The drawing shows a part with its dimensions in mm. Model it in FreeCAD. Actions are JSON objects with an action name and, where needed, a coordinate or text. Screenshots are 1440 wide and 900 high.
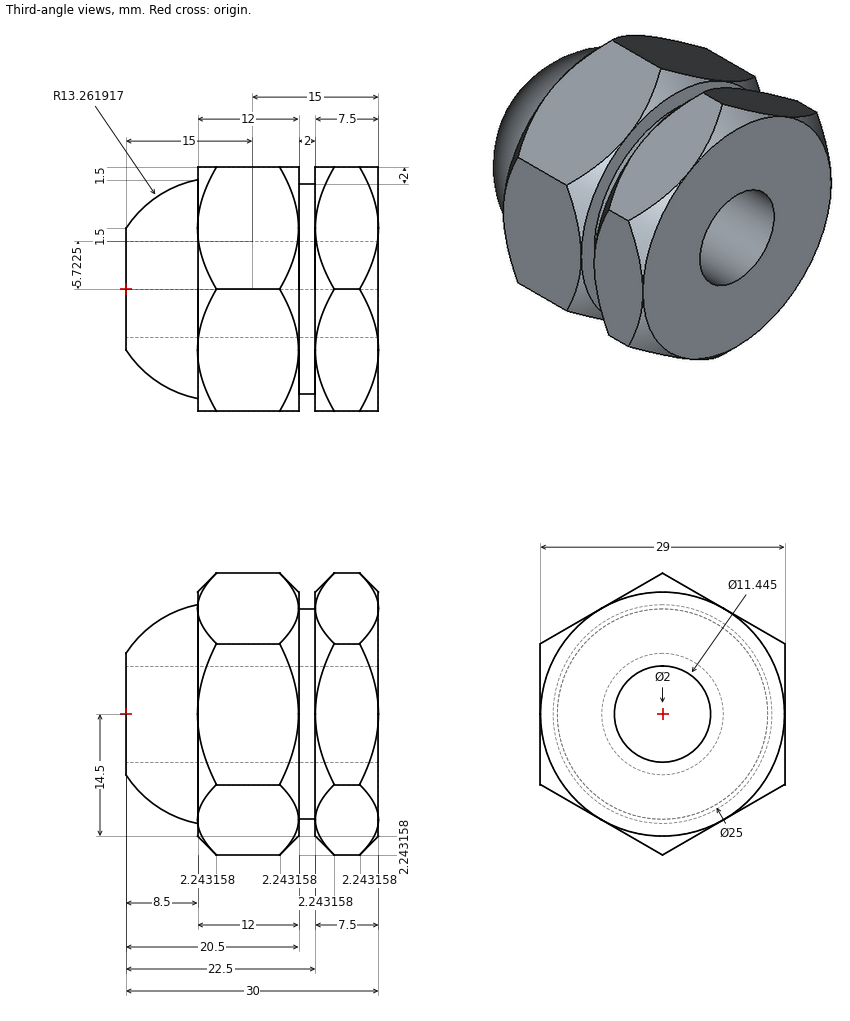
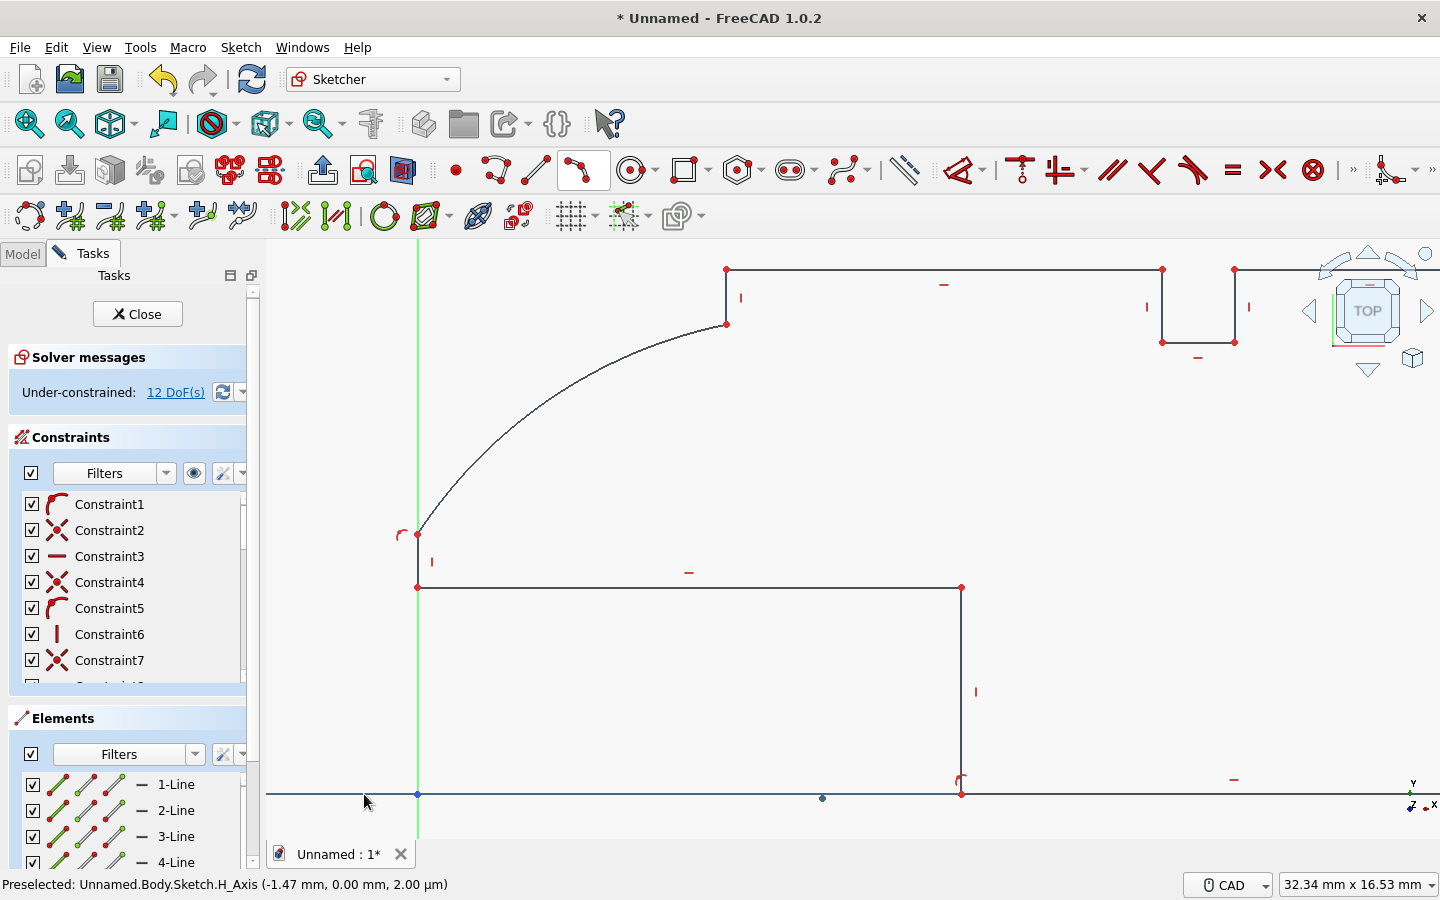
{"action": "left_click", "coordinate": [1020, 170]}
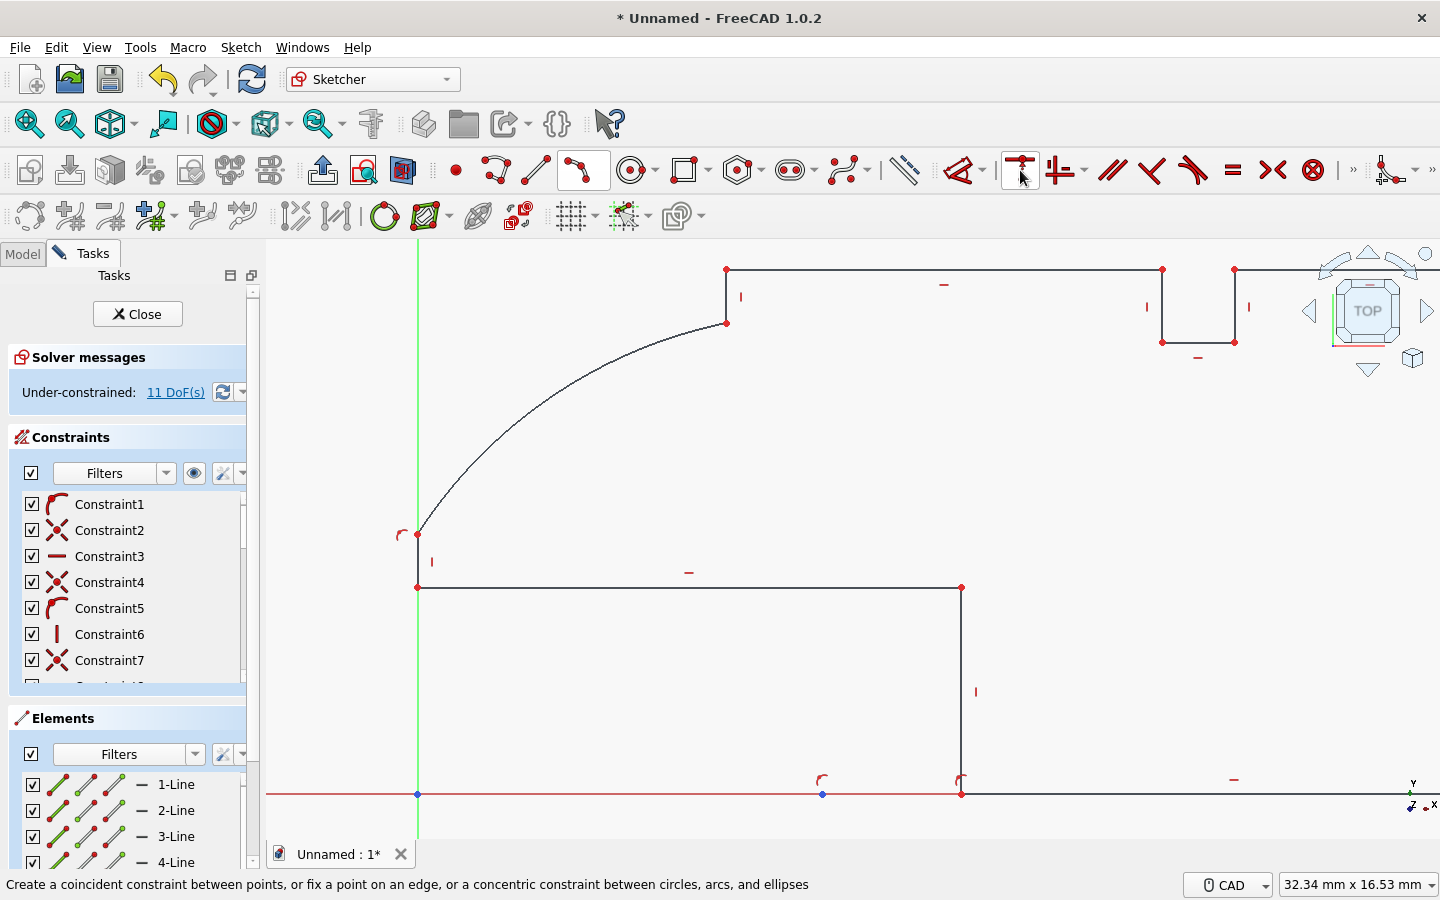
{"action": "left_click", "coordinate": [617, 359]}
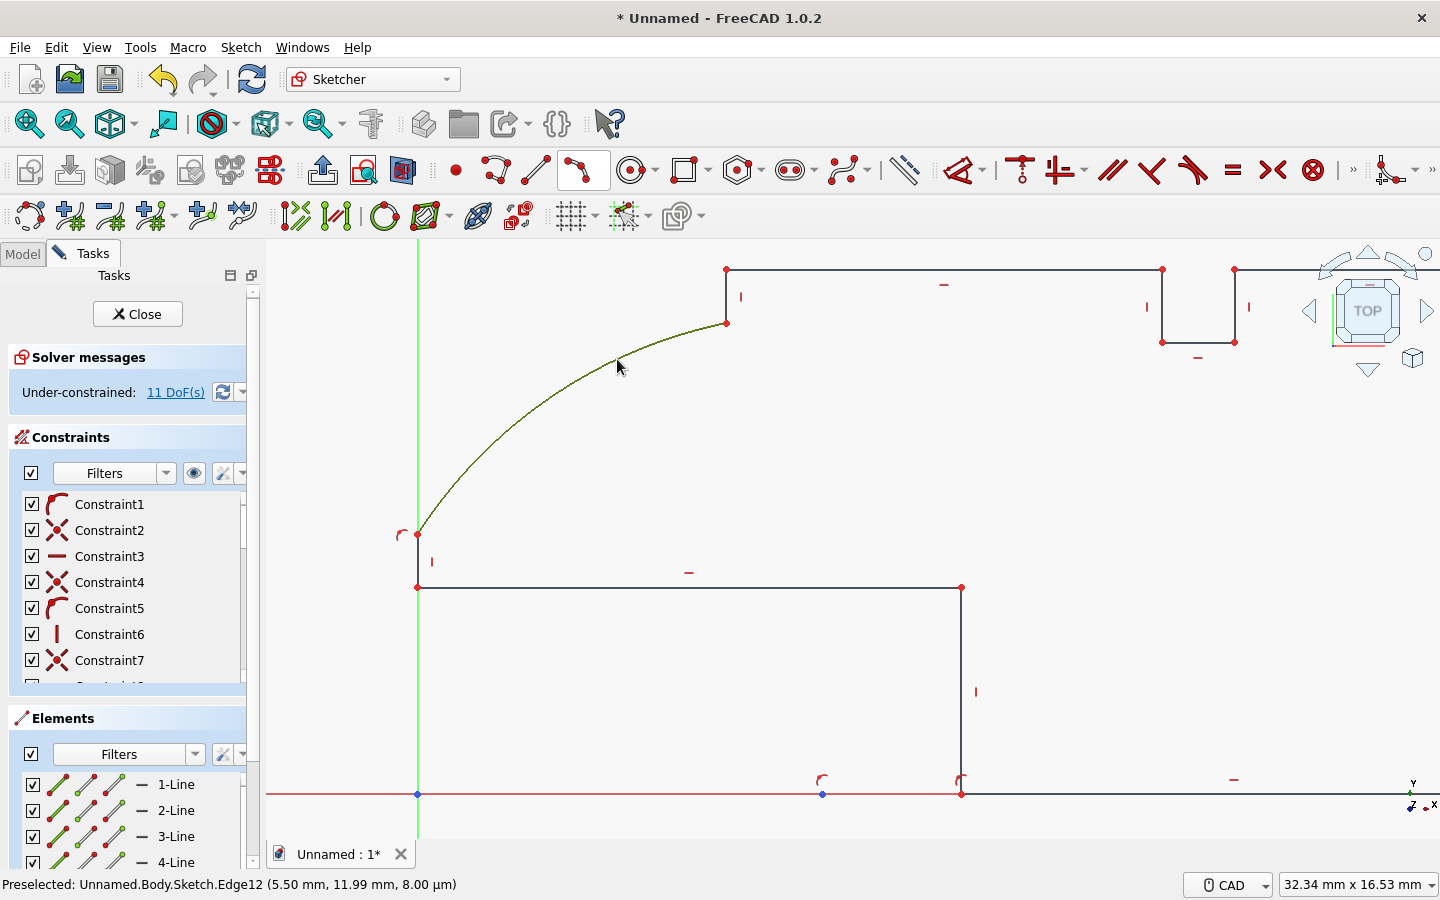
{"action": "key", "text": "k r"}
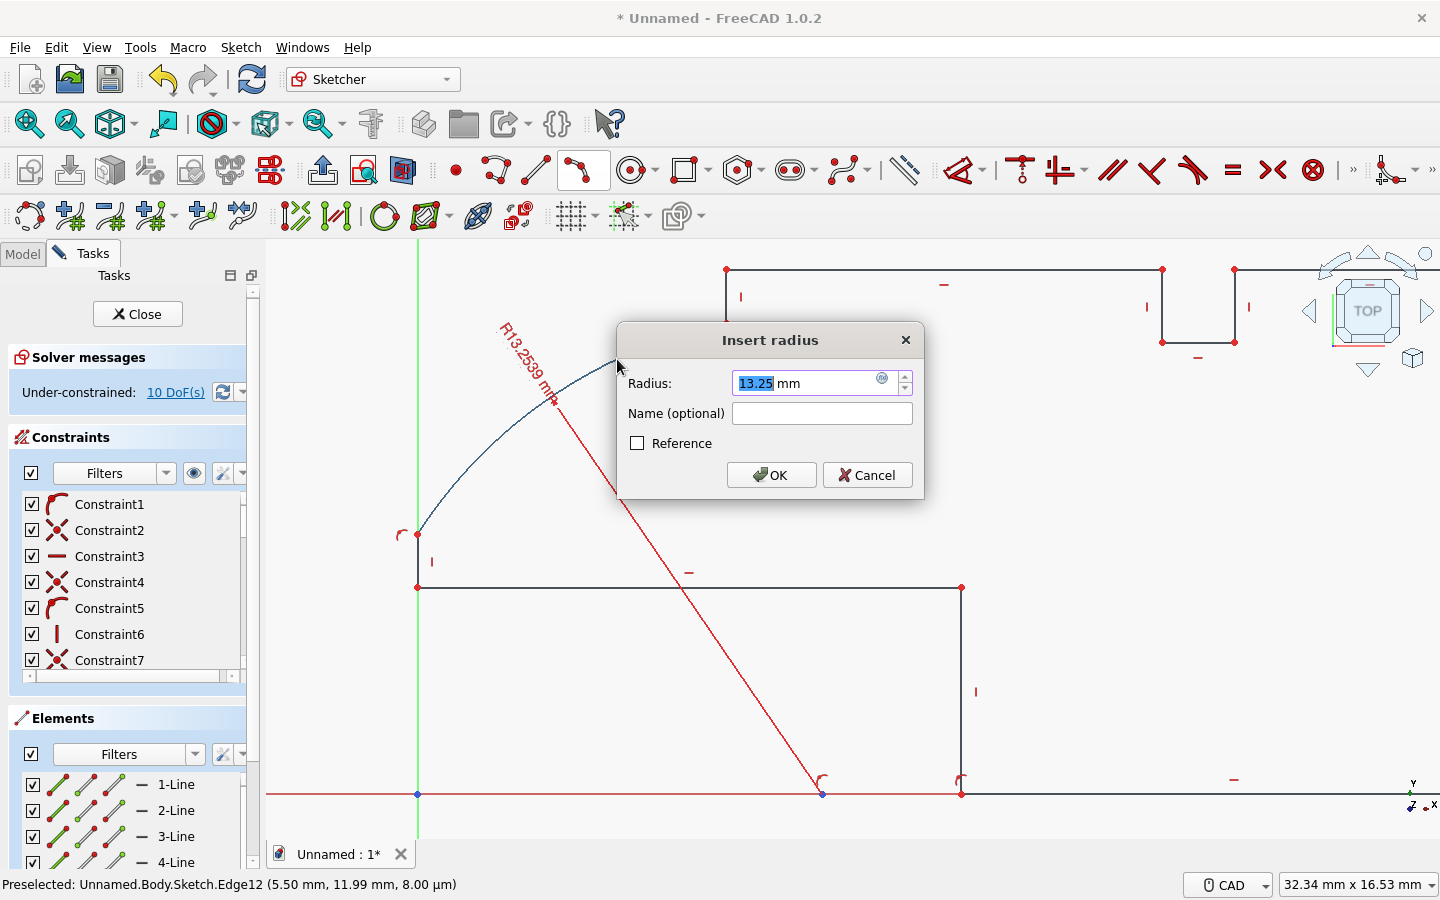
{"action": "type", "text": "13.261917"}
{"action": "key", "text": "Return"}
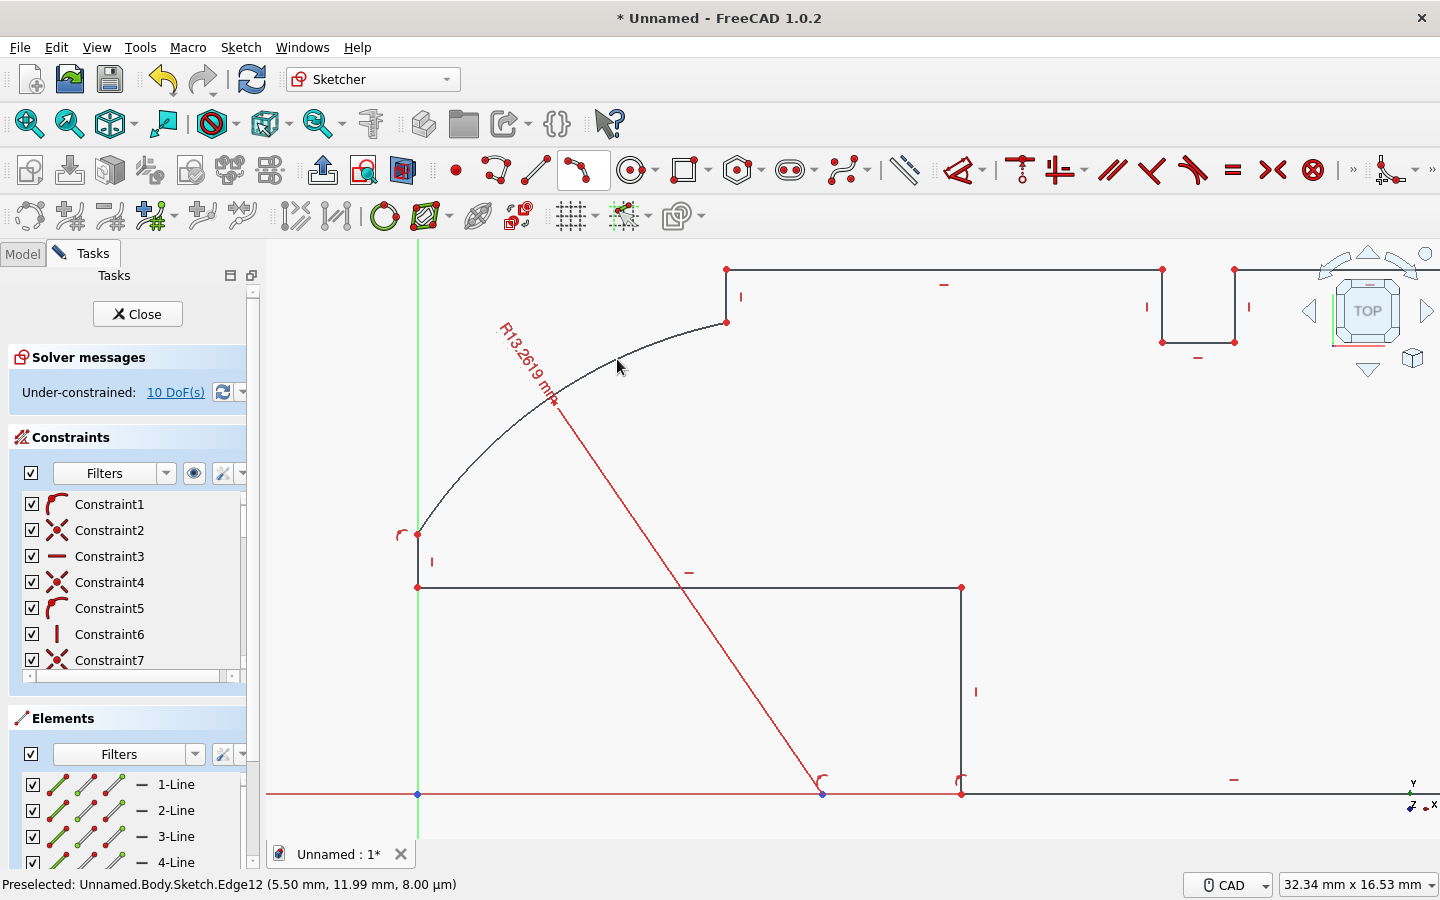
{"action": "left_click", "coordinate": [1235, 292]}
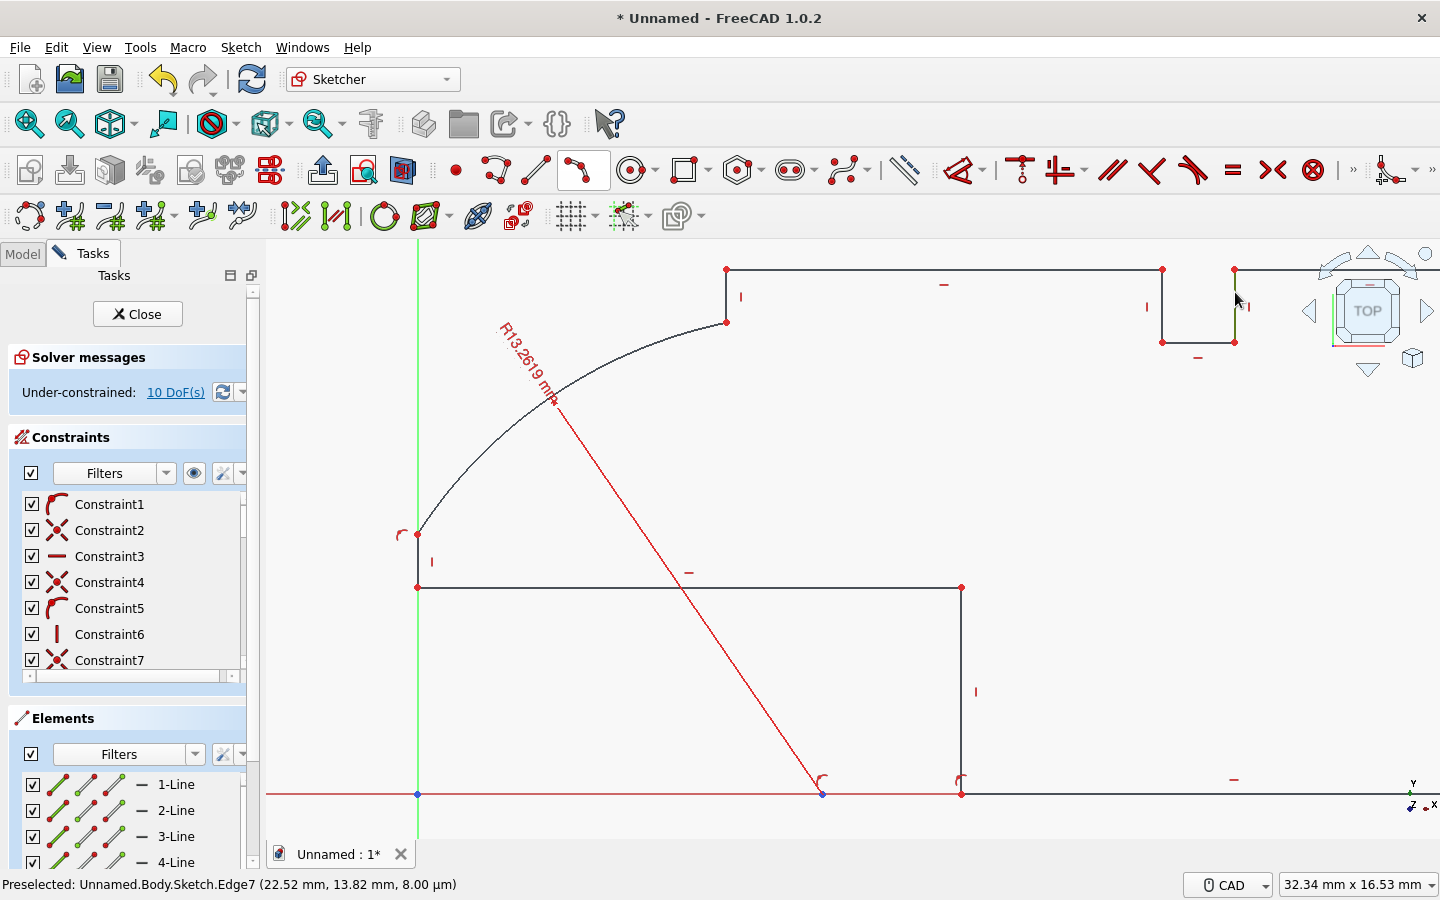
{"action": "key", "text": "i"}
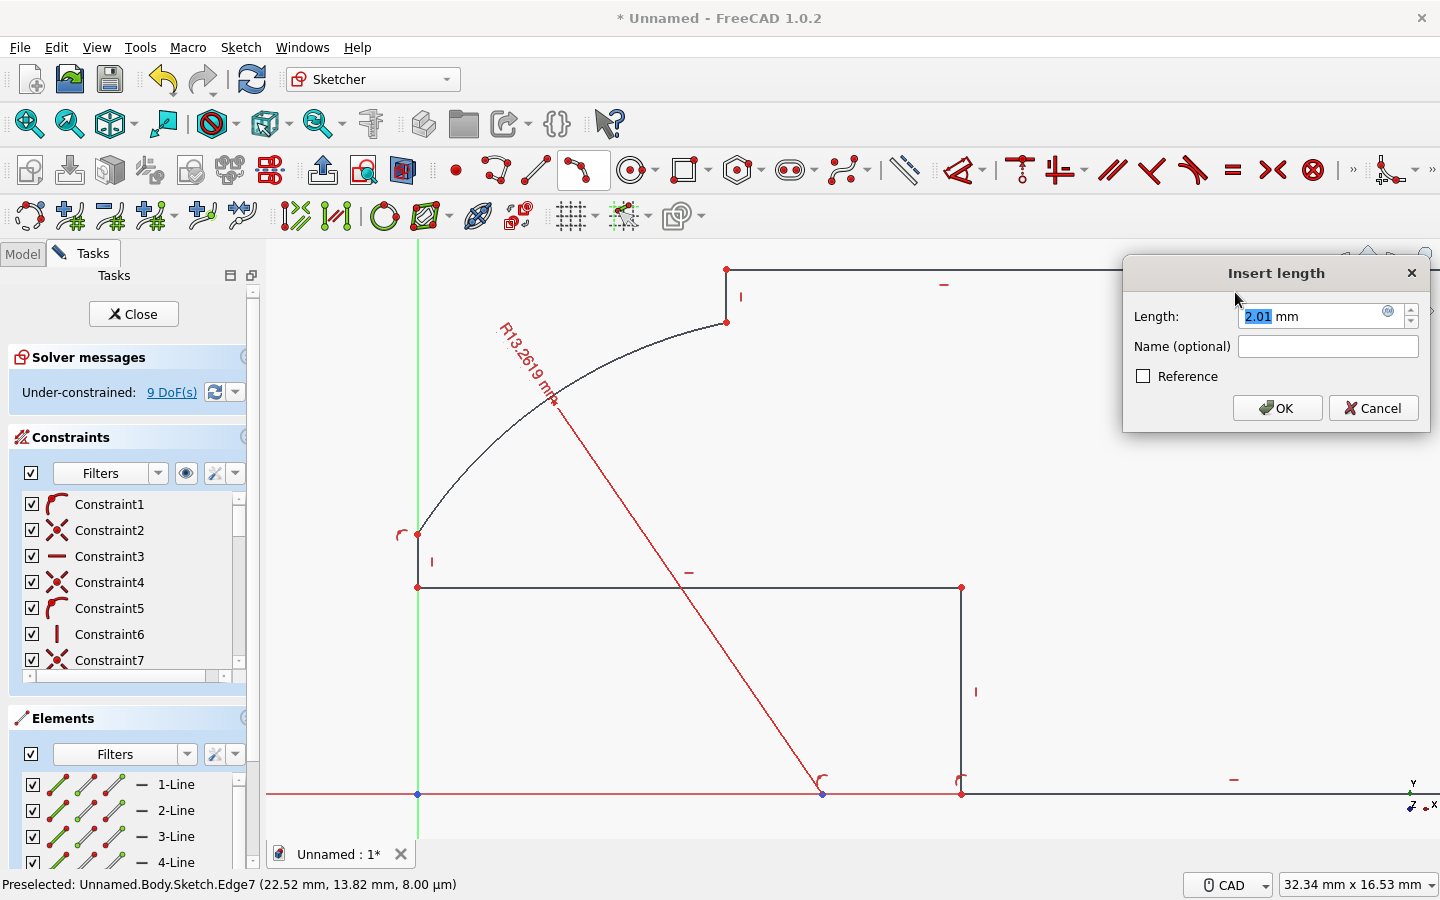
{"action": "type", "text": "2"}
{"action": "key", "text": "Return"}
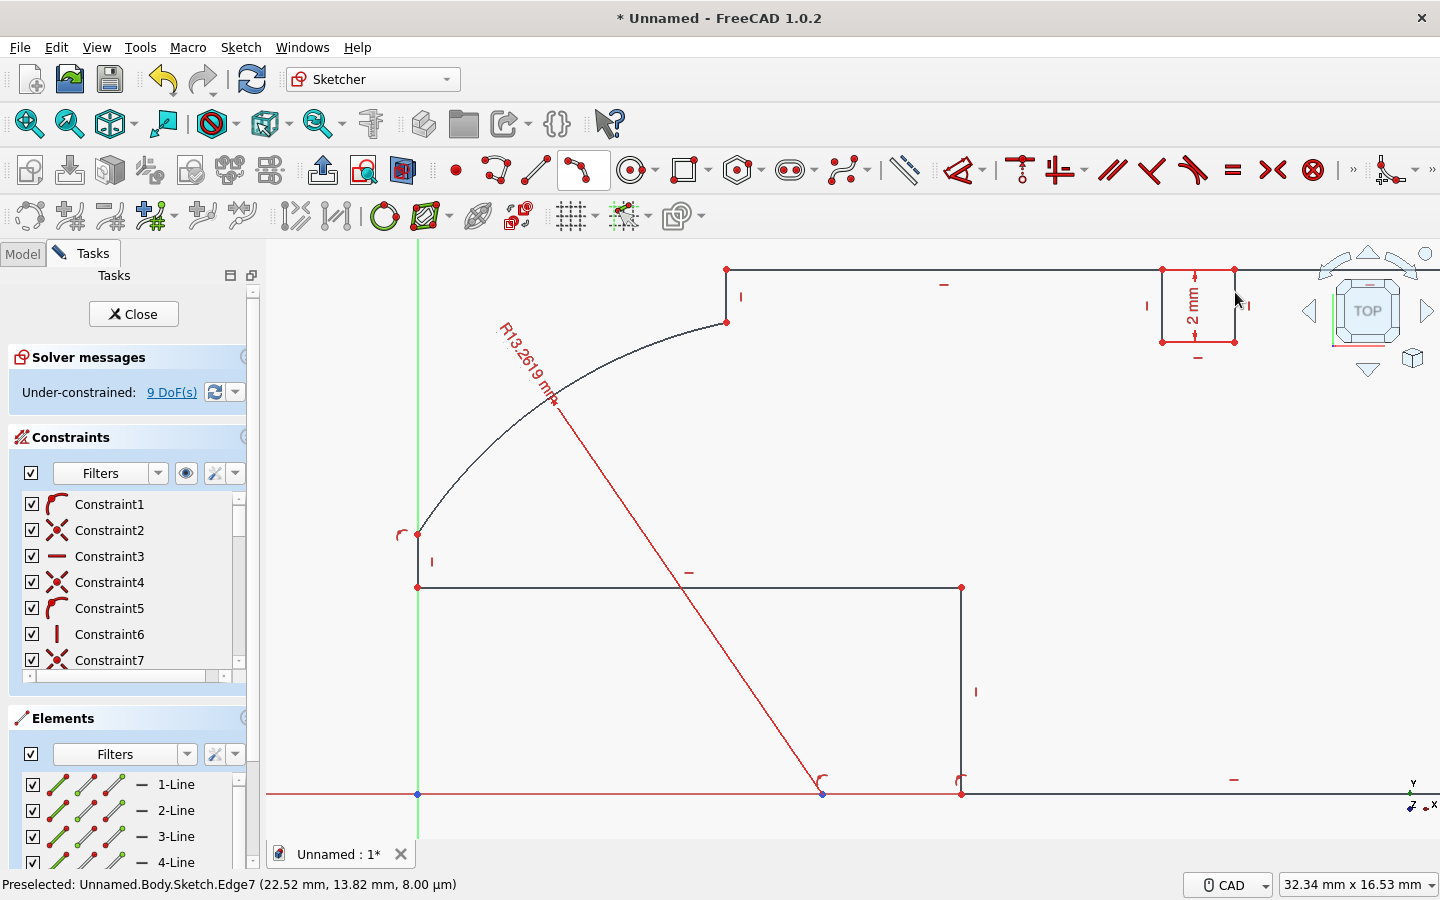
{"action": "left_click", "coordinate": [1213, 342]}